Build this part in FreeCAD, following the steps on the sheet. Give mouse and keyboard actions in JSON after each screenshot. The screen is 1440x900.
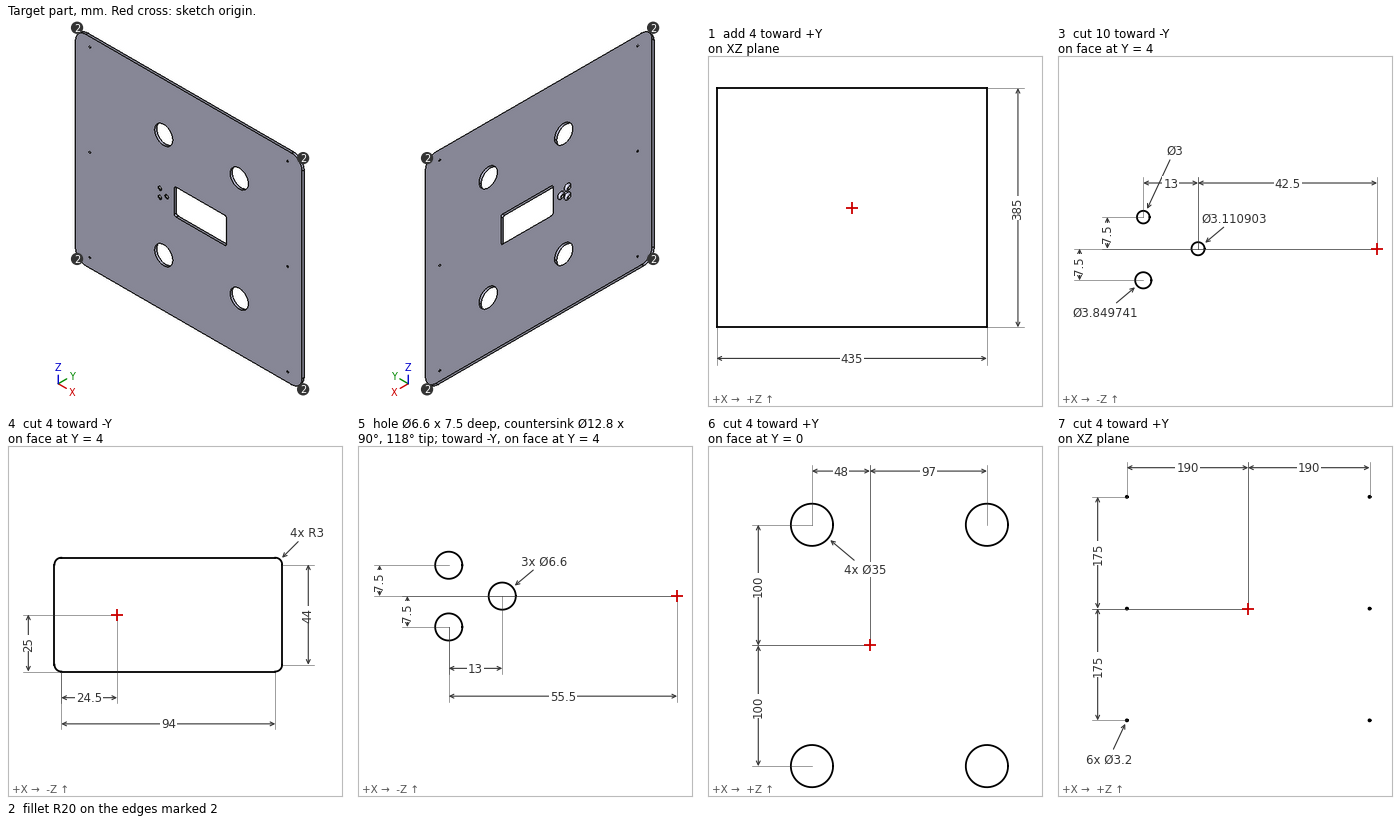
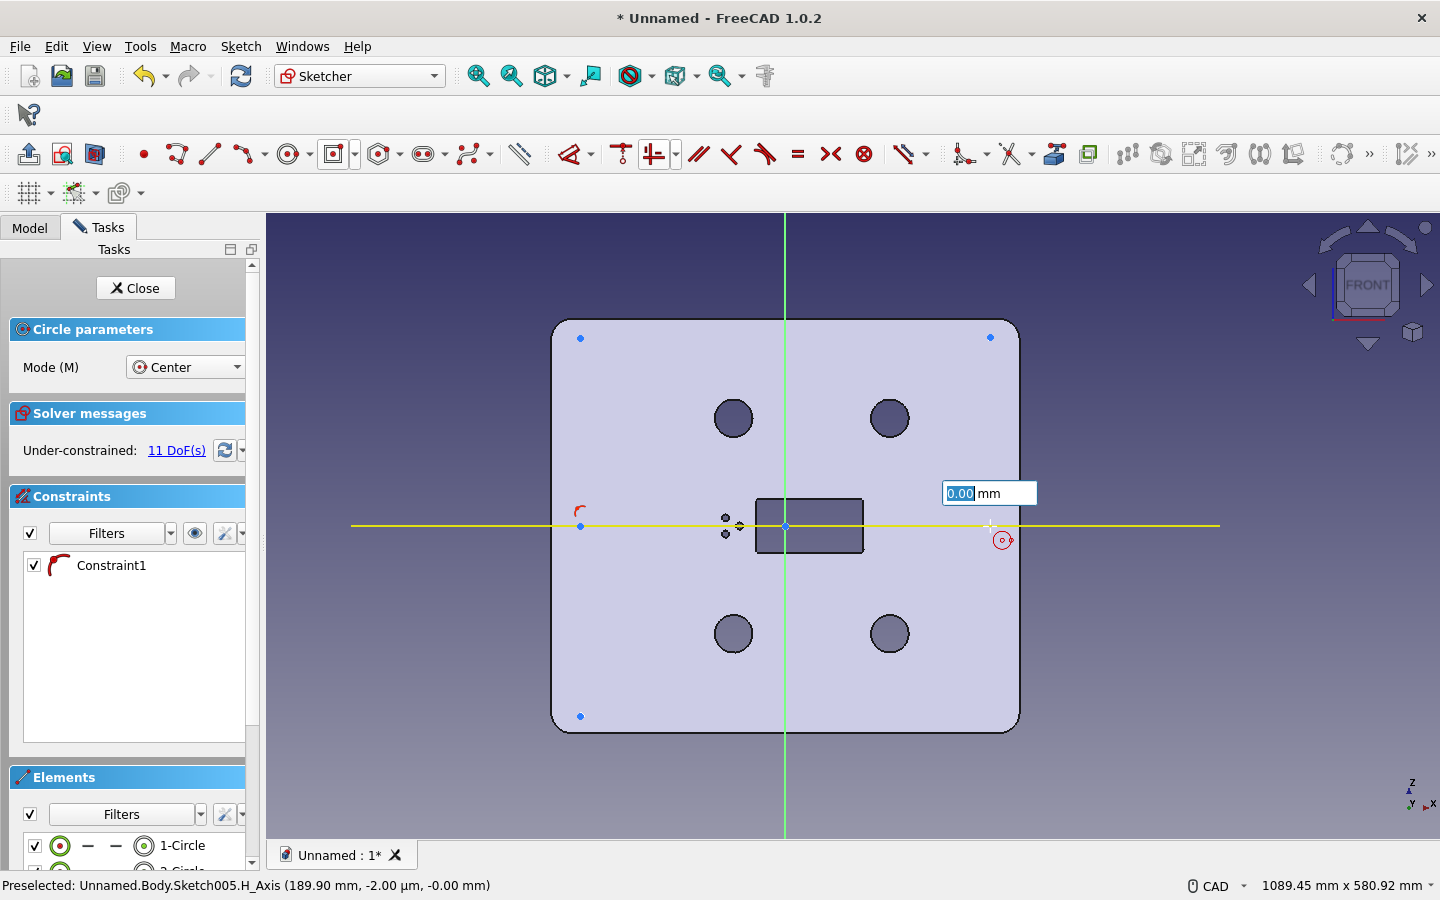
{"action": "scroll", "coordinate": [990, 528], "scroll_direction": "up", "scroll_amount": 12}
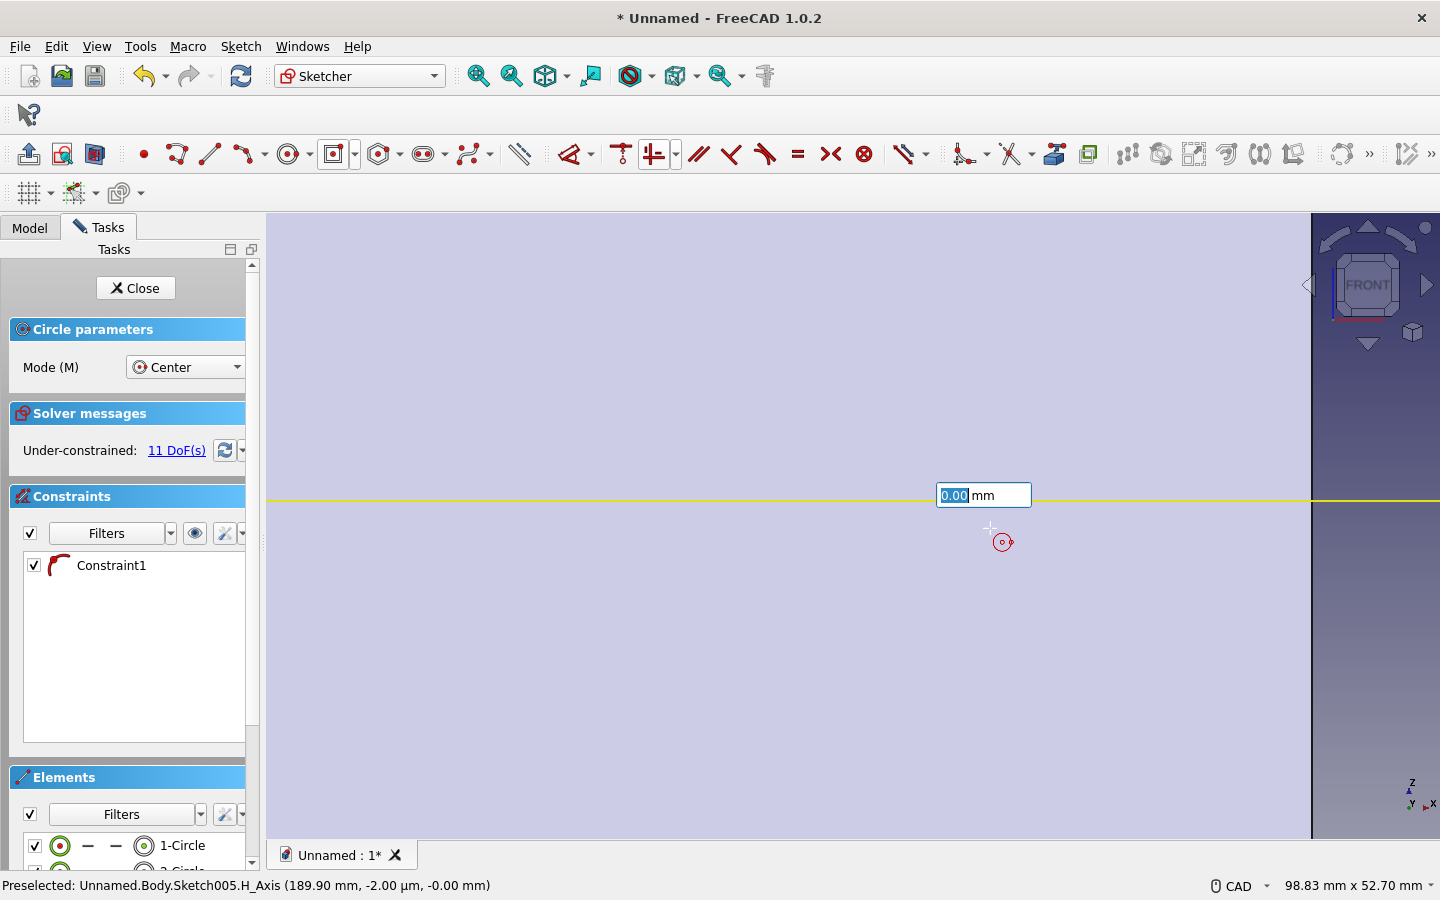
{"action": "left_click", "coordinate": [979, 519]}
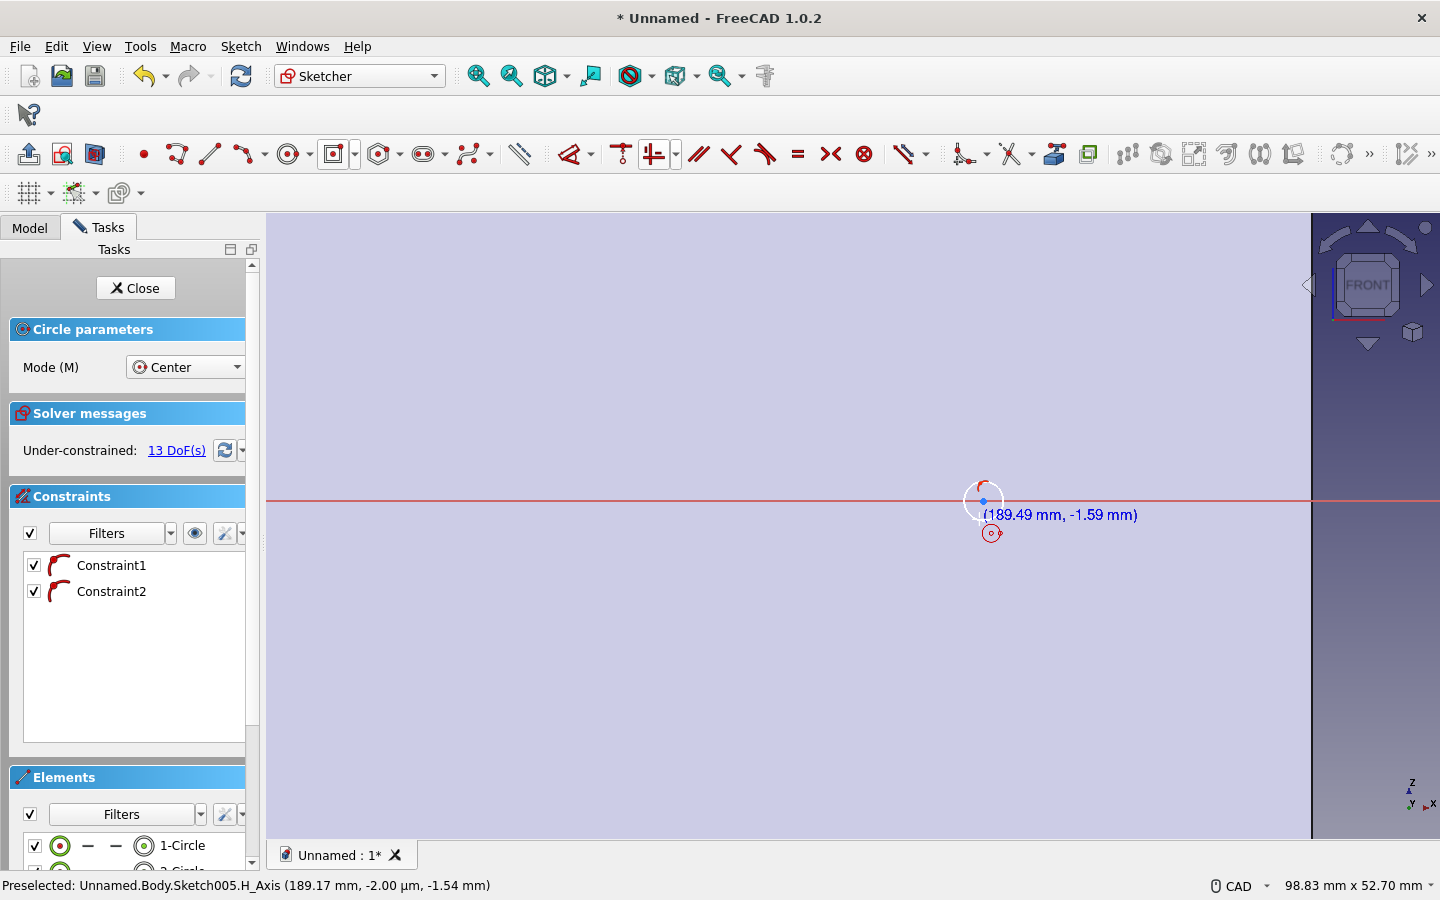
{"action": "scroll", "coordinate": [990, 528], "scroll_direction": "down", "scroll_amount": 12}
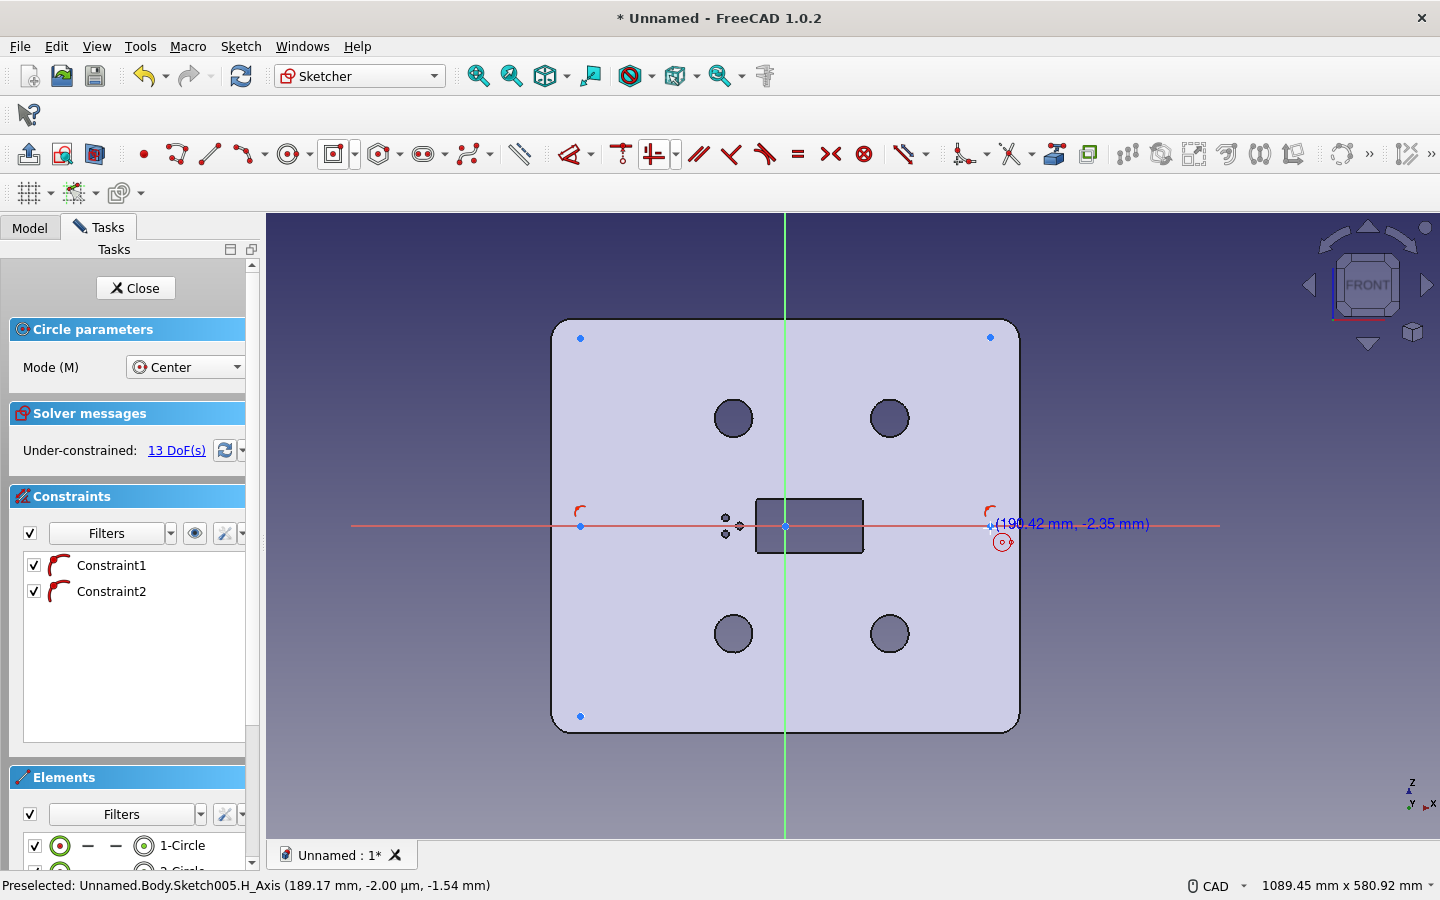
{"action": "scroll", "coordinate": [990, 715], "scroll_direction": "up", "scroll_amount": 13}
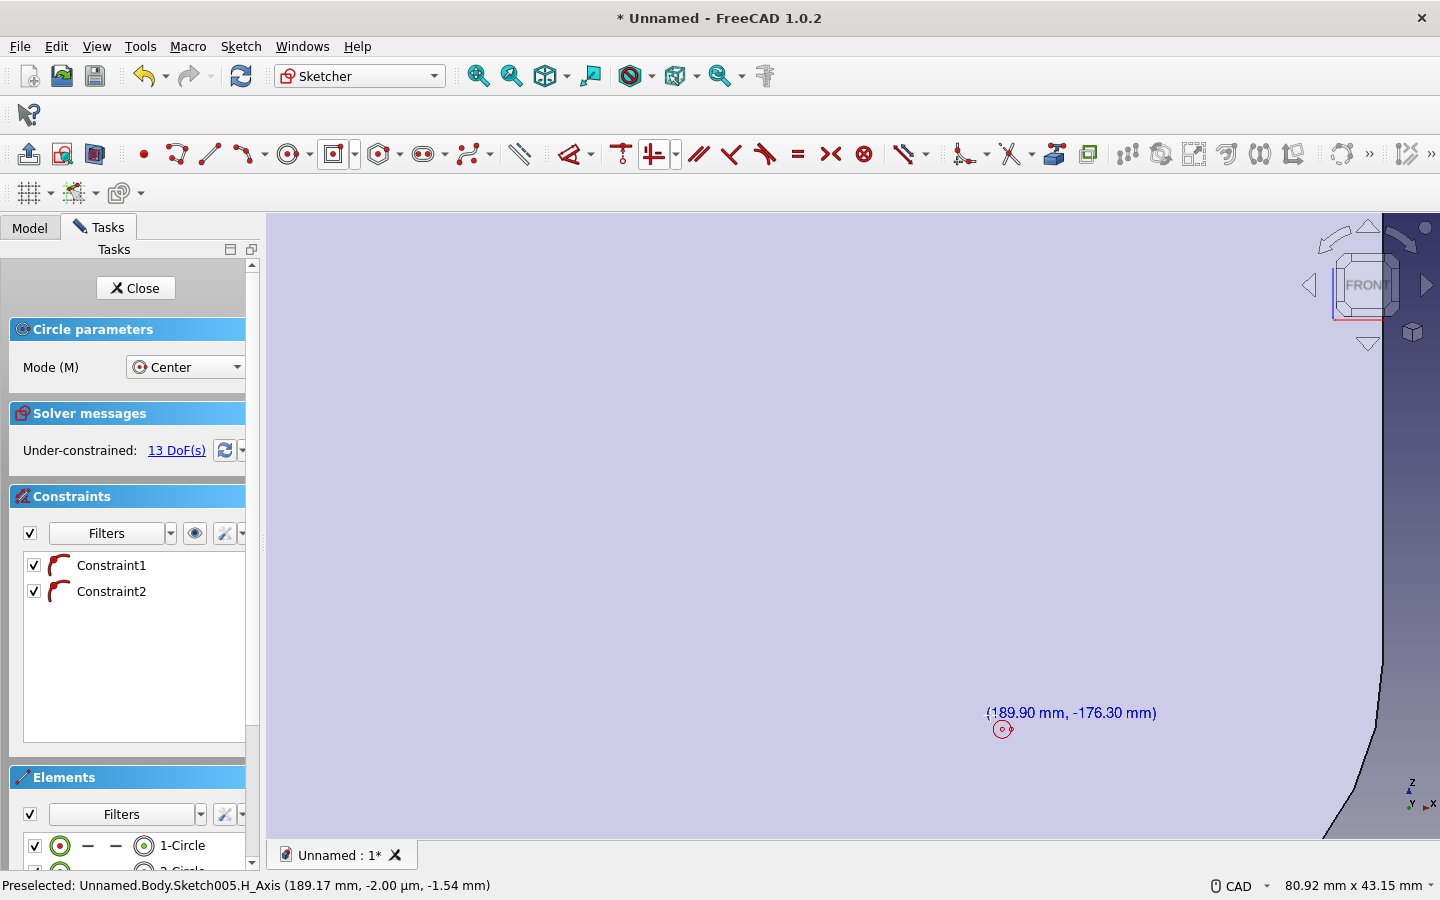
{"action": "scroll", "coordinate": [990, 716], "scroll_direction": "down", "scroll_amount": 13}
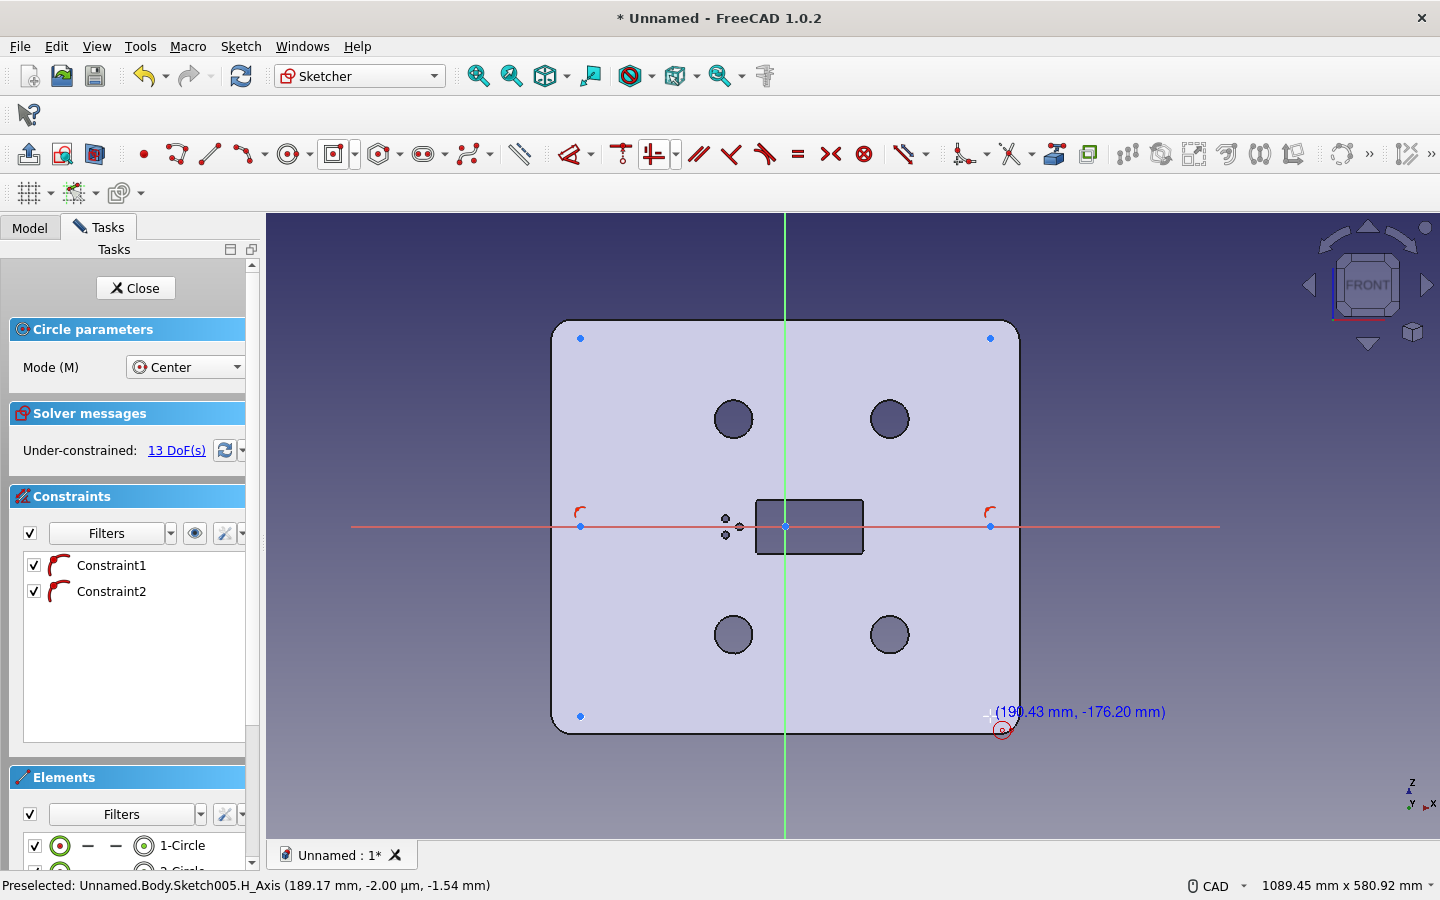
{"action": "left_click", "coordinate": [990, 716]}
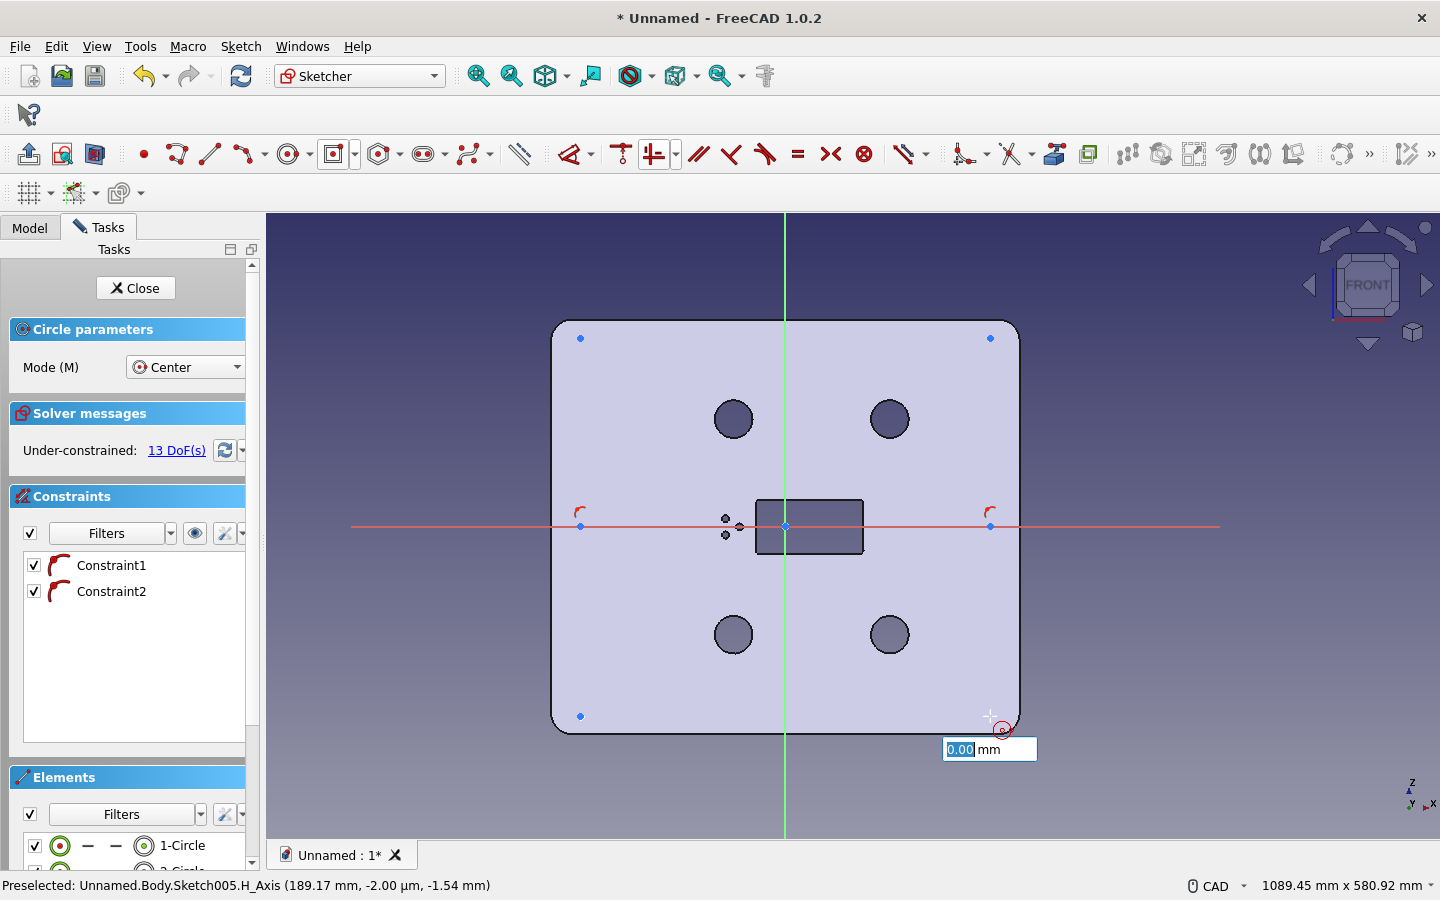
{"action": "scroll", "coordinate": [991, 714], "scroll_direction": "up", "scroll_amount": 12}